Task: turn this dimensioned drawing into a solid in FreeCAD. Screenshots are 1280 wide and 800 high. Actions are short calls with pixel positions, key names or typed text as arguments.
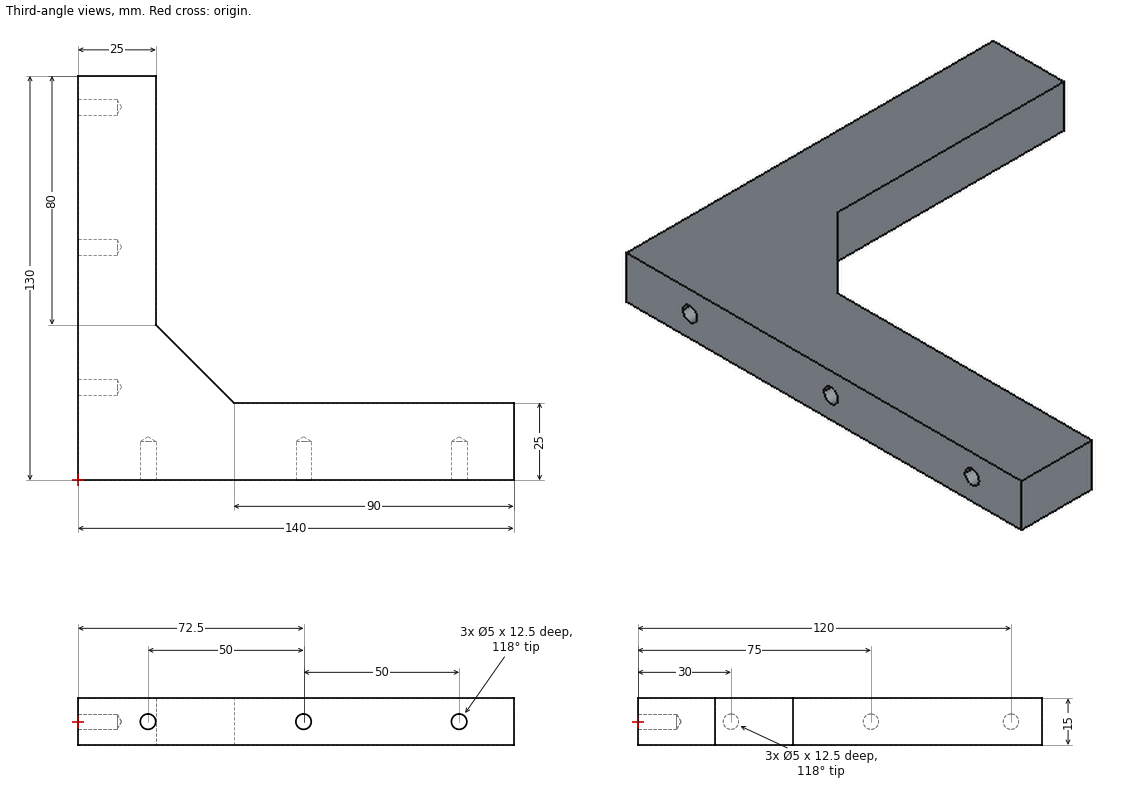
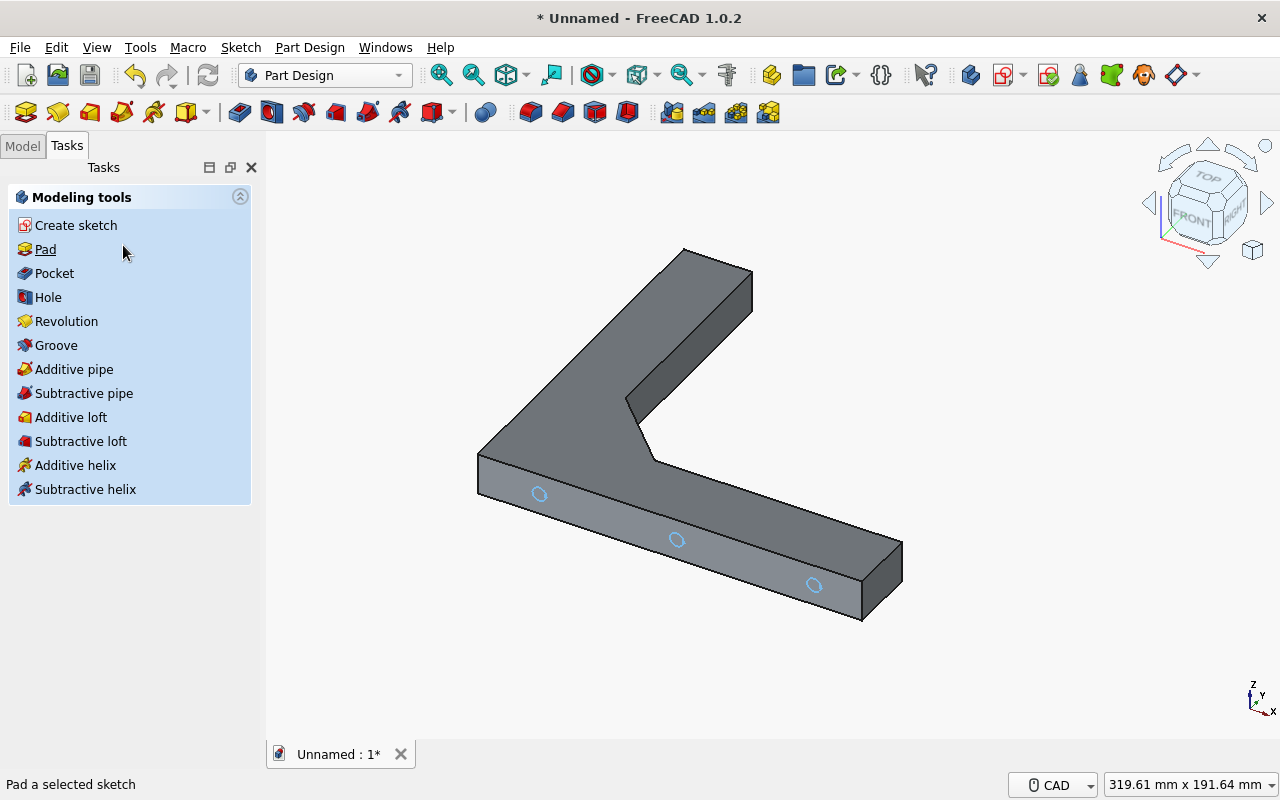
click(272, 112)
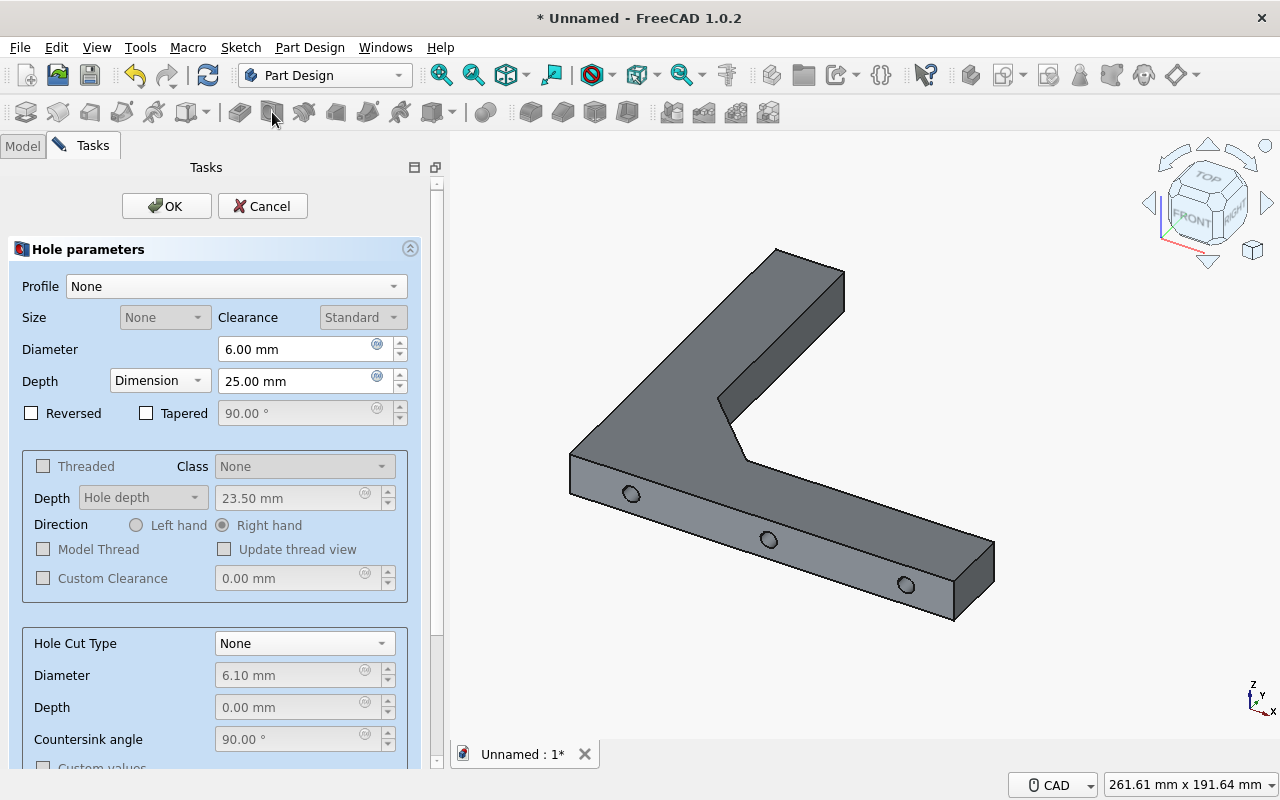
triple_click(305, 349)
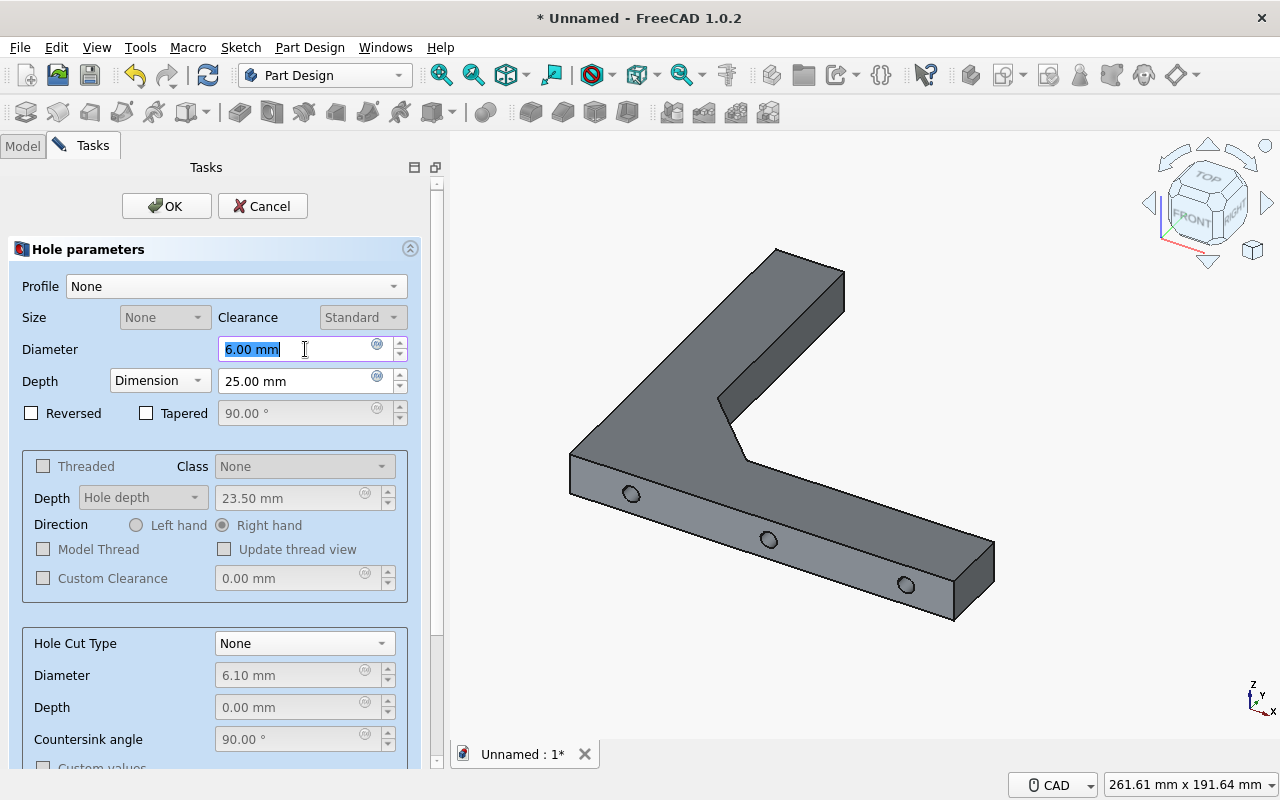
text(5)
key(Tab)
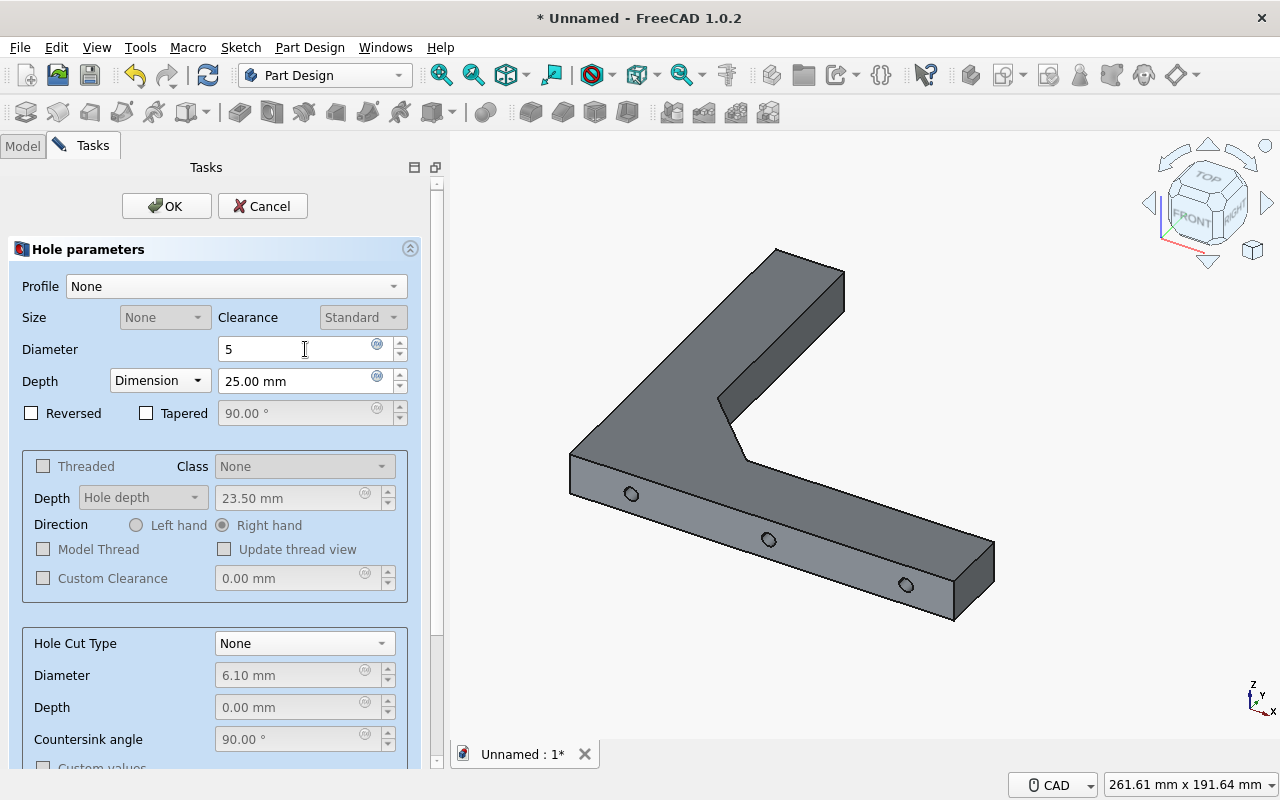
triple_click(305, 381)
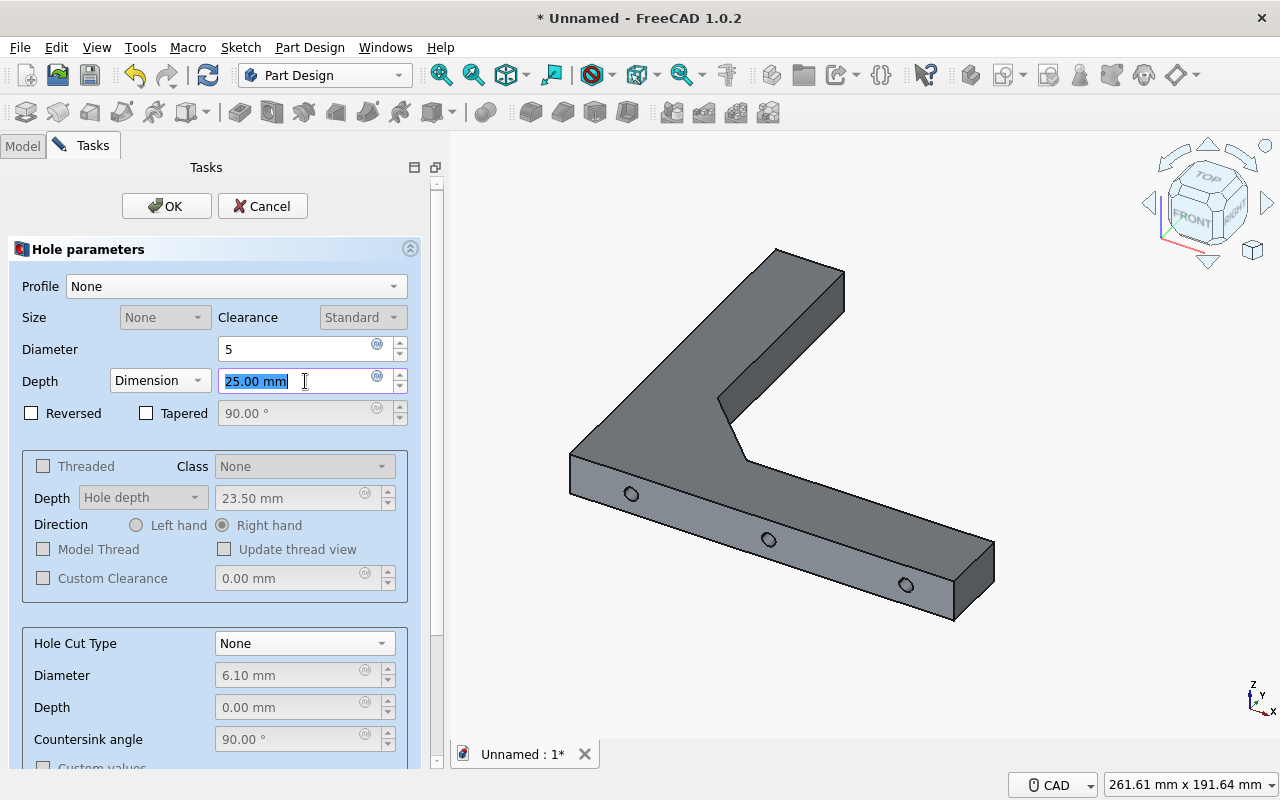
text(12.5)
key(Tab)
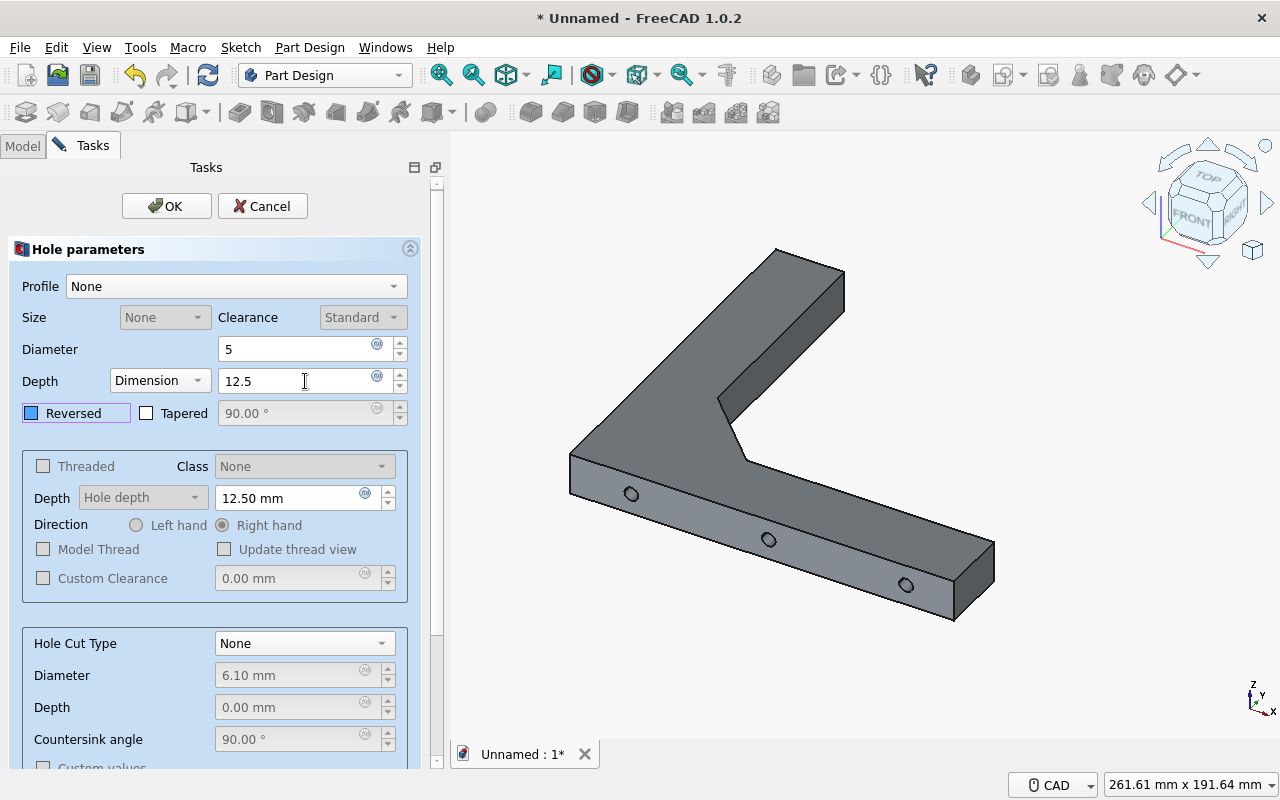
click(167, 206)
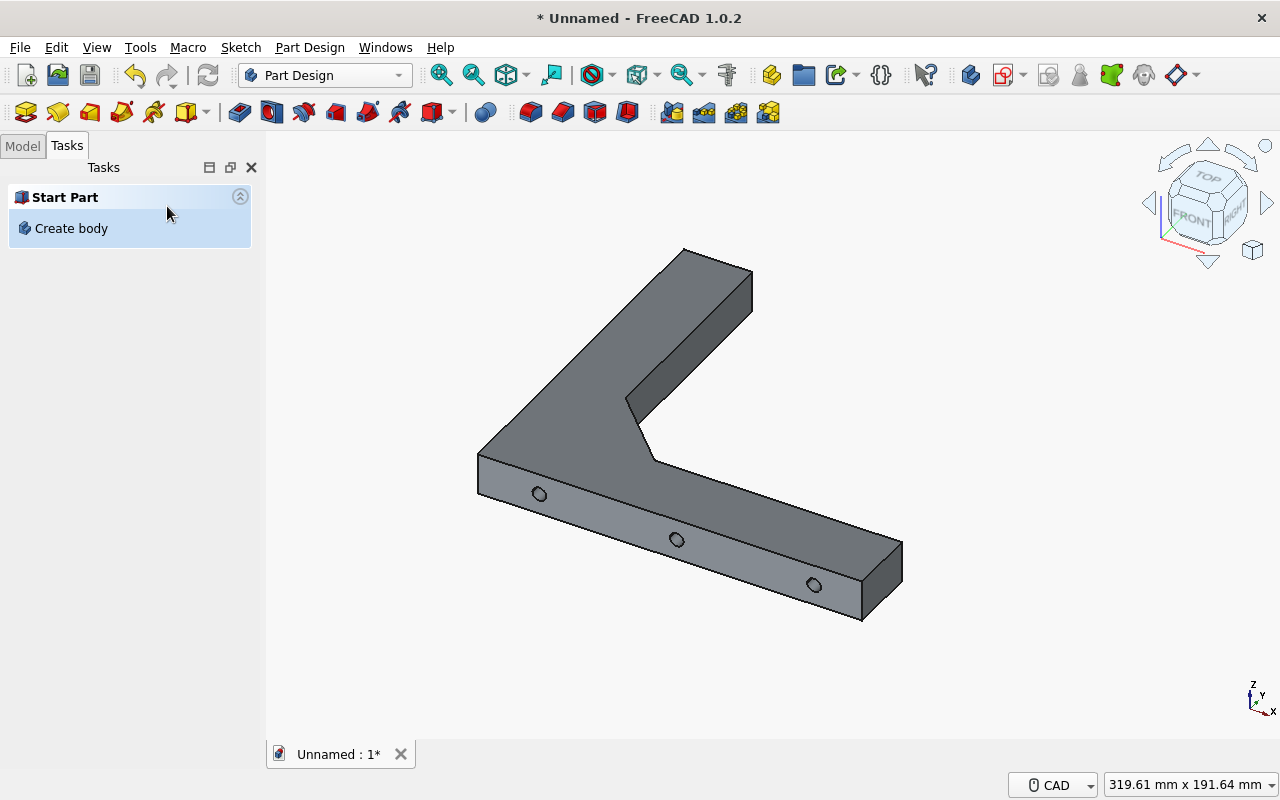
click(1004, 76)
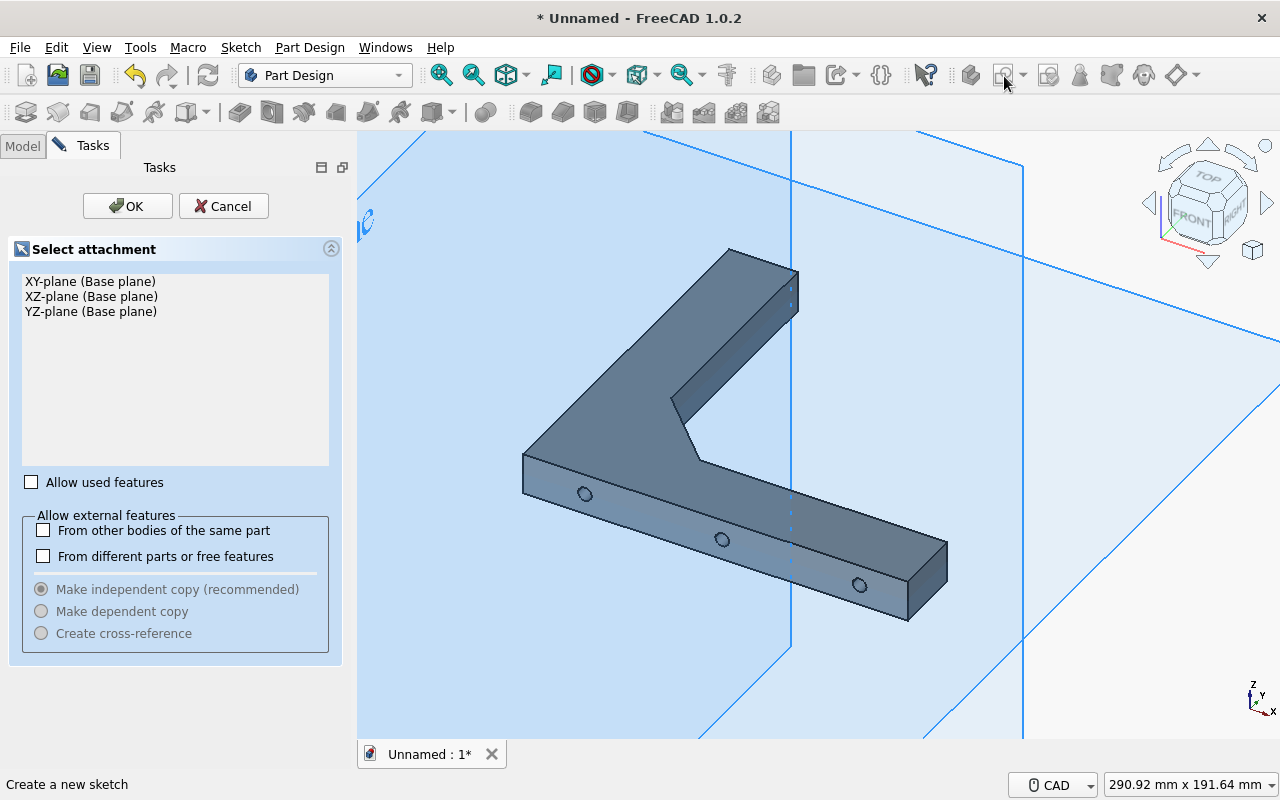
click(82, 312)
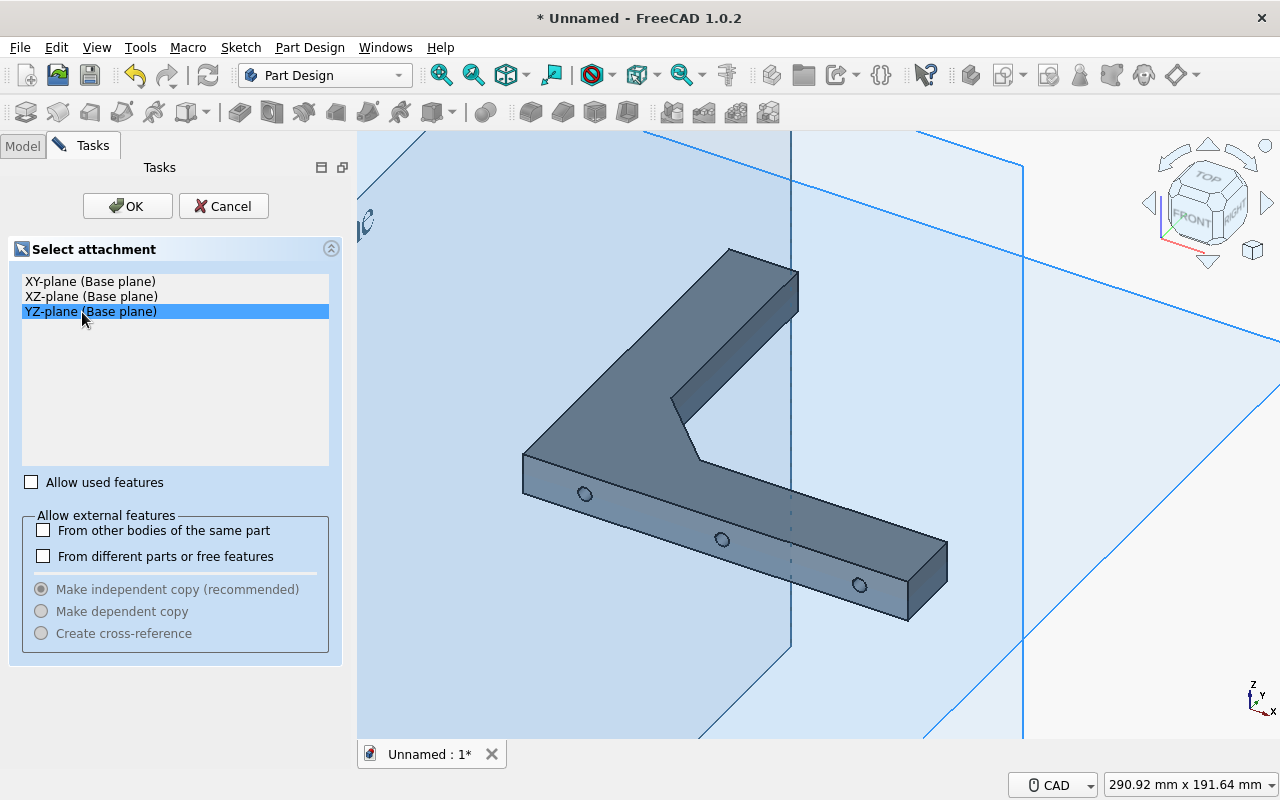
click(128, 206)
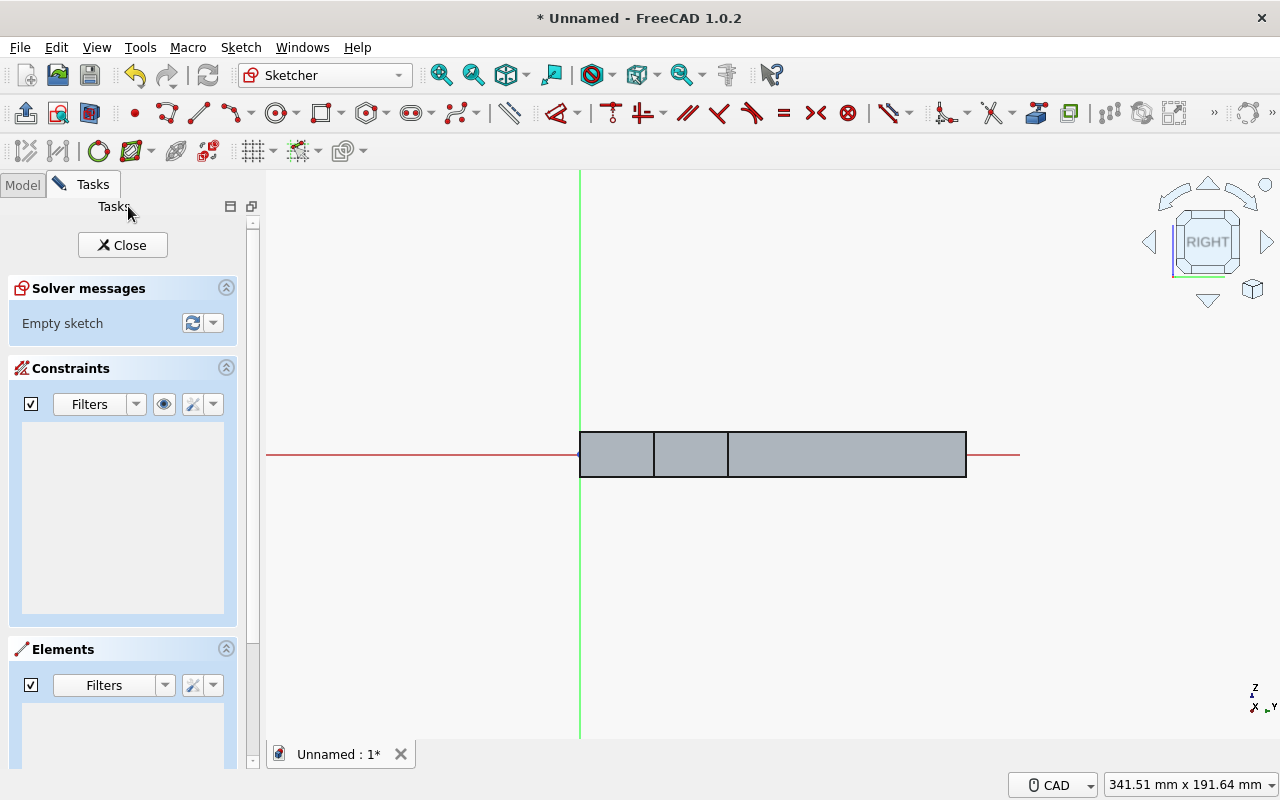
click(90, 114)